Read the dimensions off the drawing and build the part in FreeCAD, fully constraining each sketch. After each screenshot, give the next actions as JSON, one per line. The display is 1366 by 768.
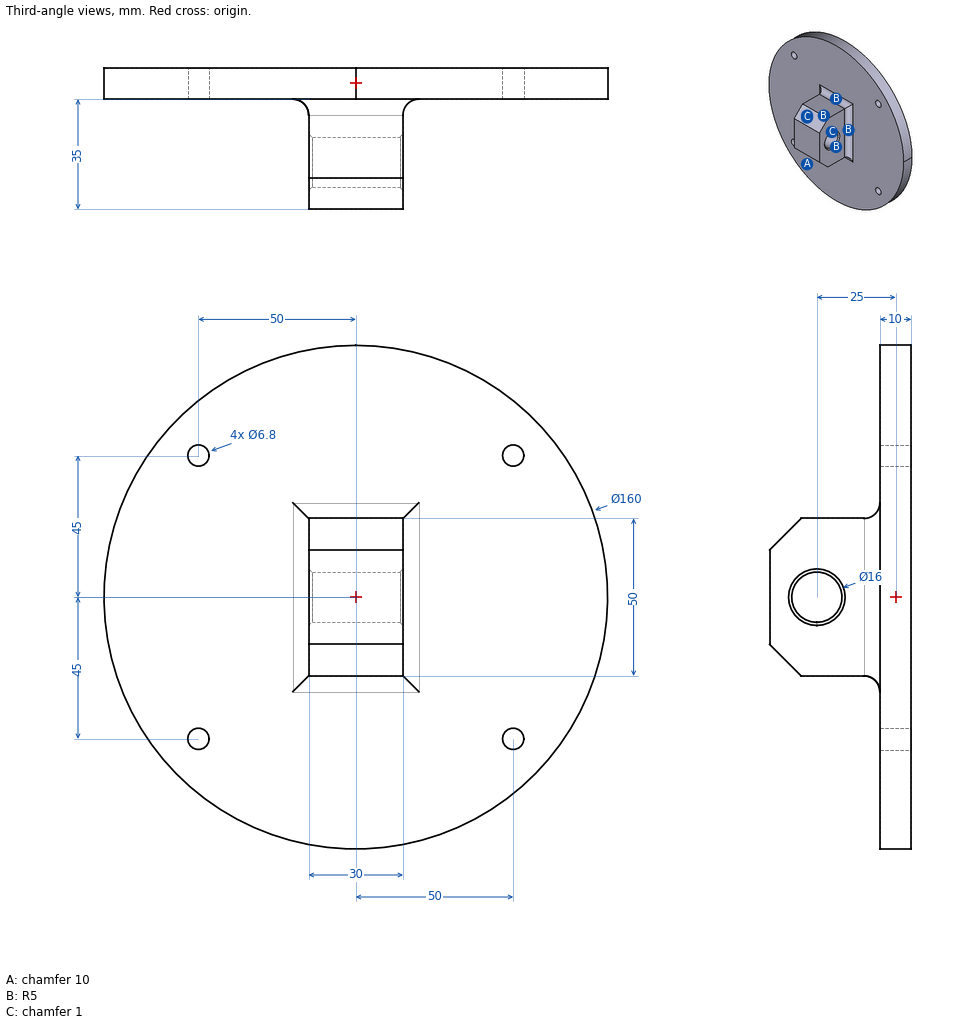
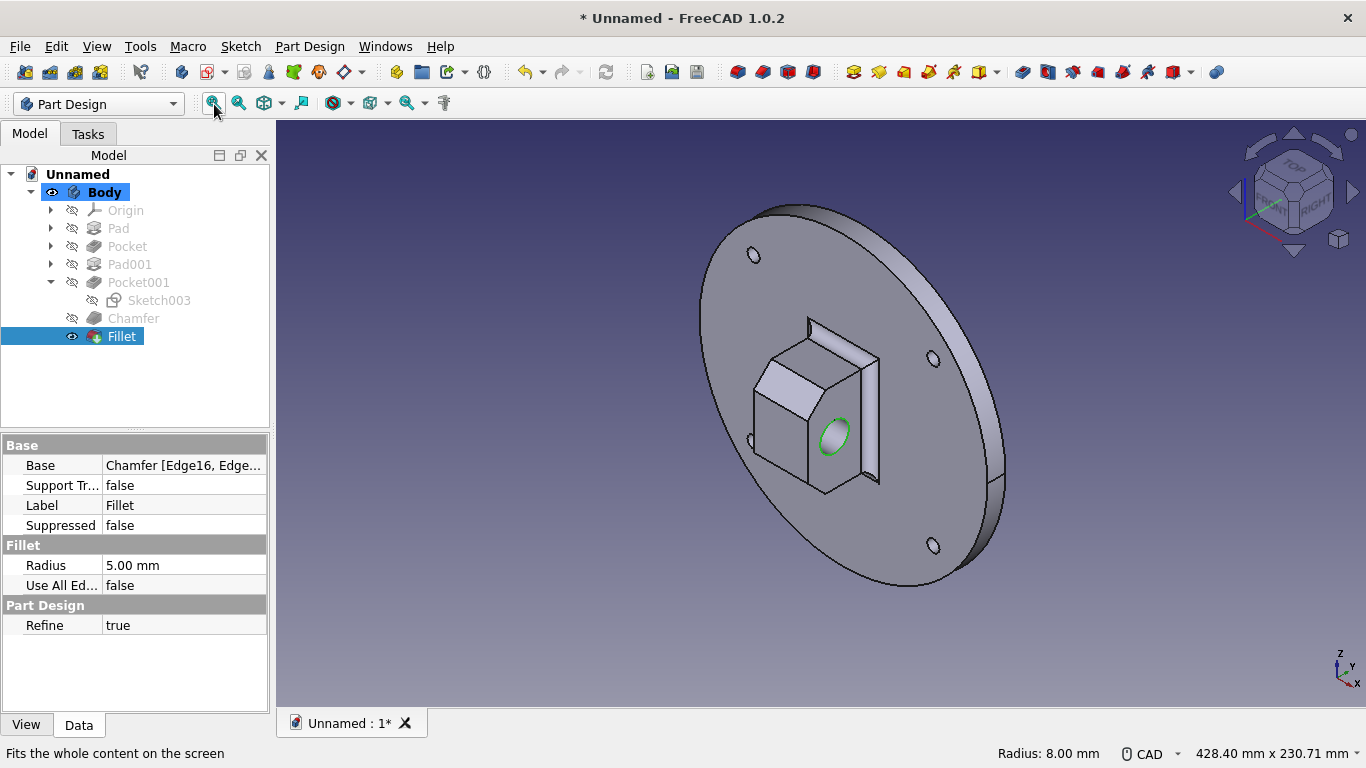
{"action": "key", "text": "1"}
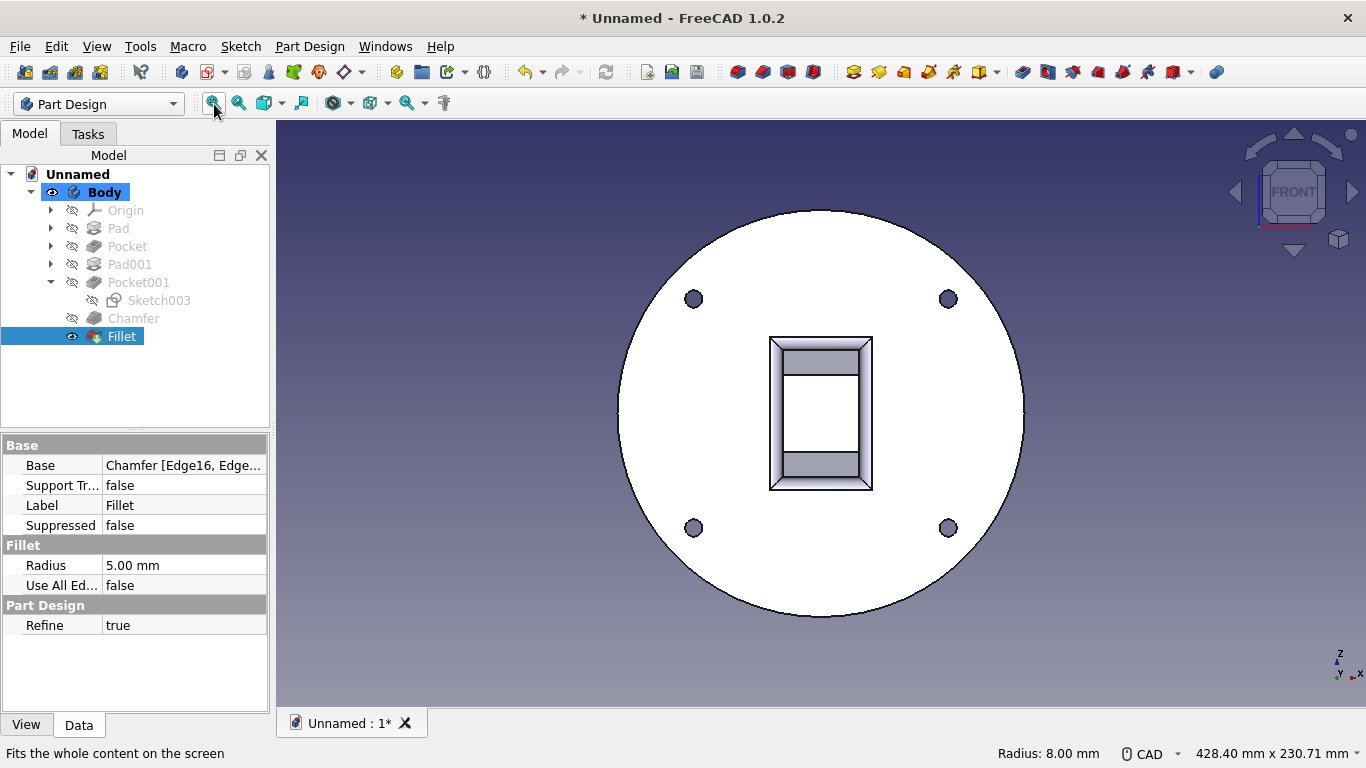
{"action": "key", "text": "3"}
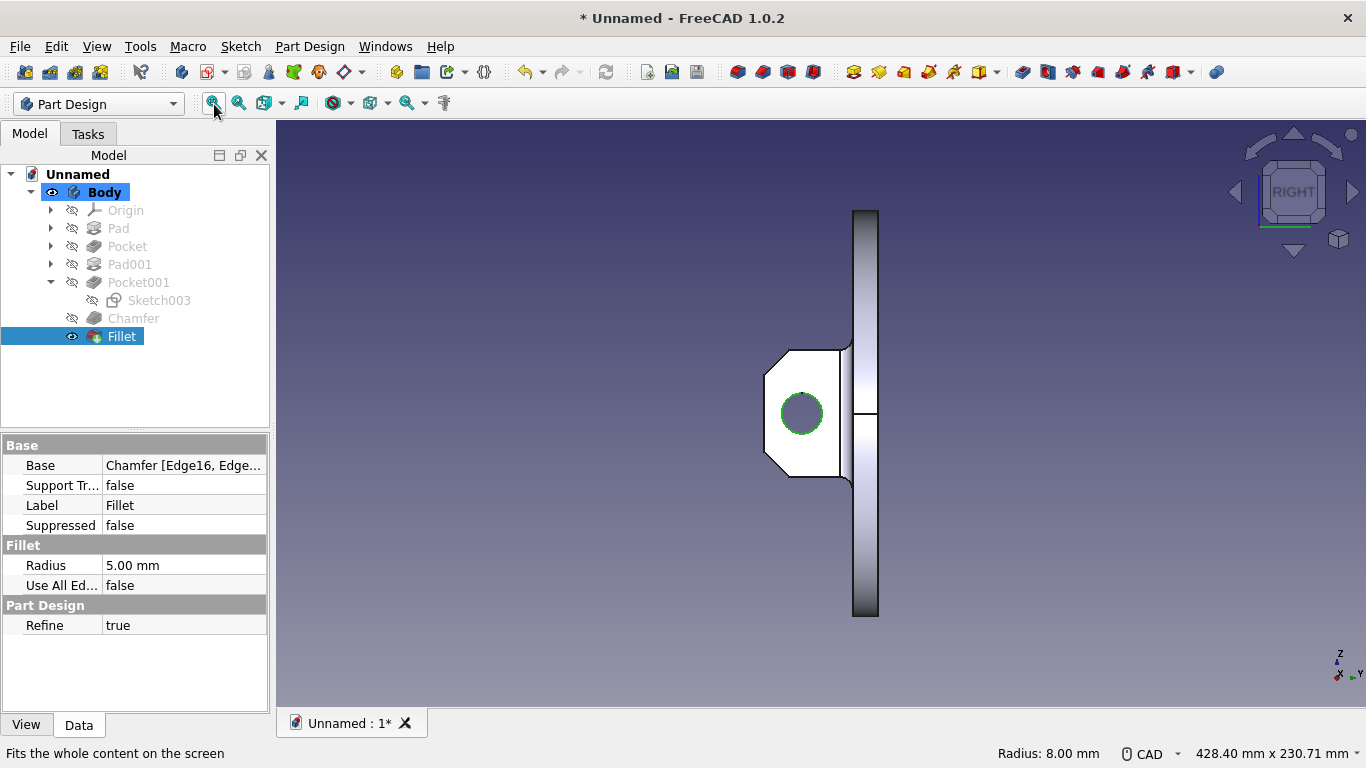
{"action": "key", "text": "5"}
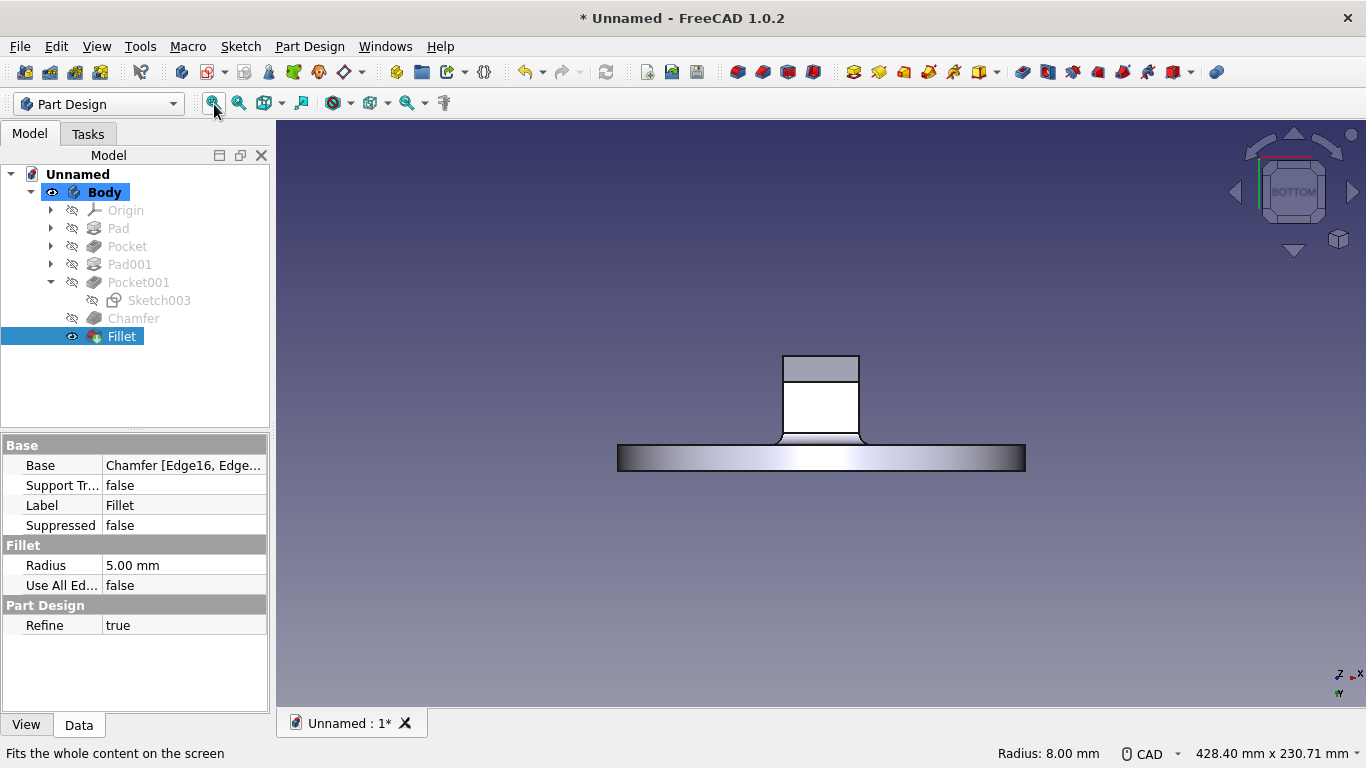
{"action": "left_click", "coordinate": [214, 104]}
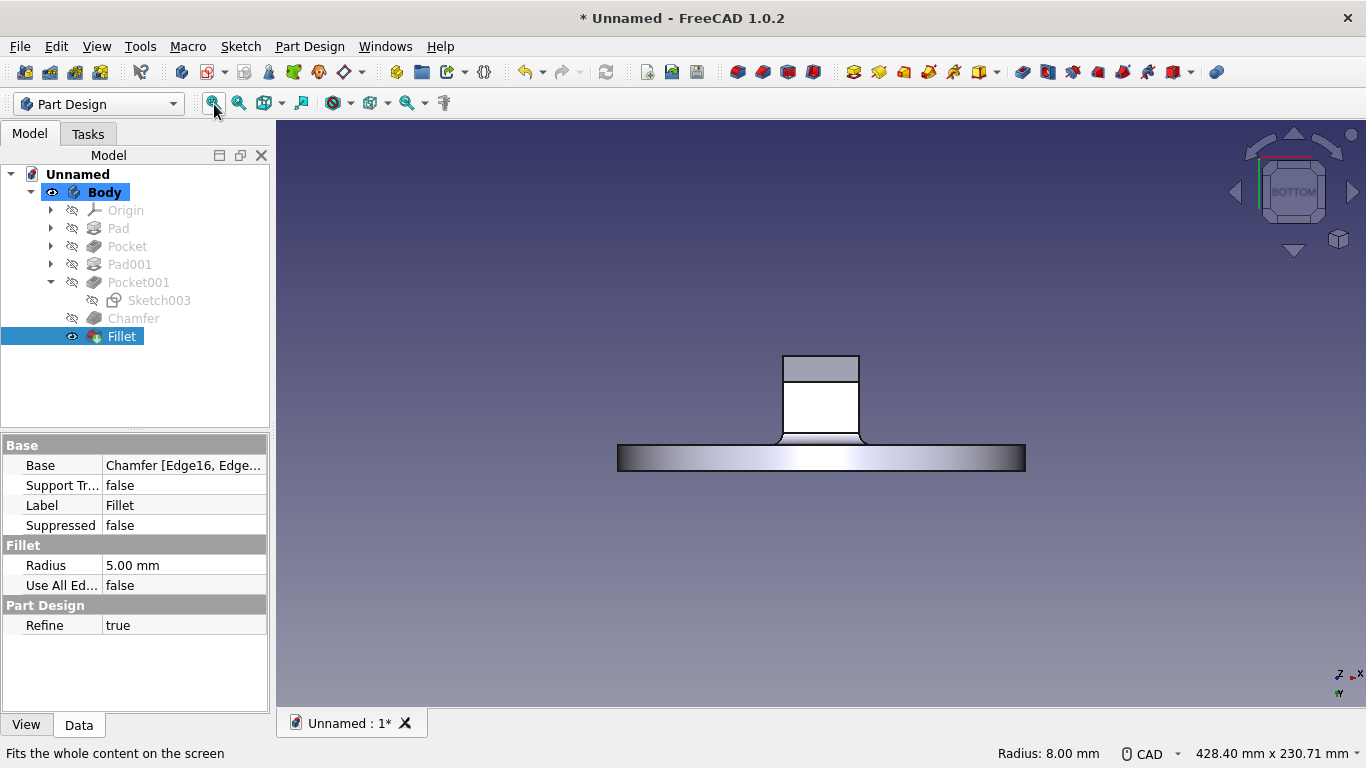
{"action": "key", "text": "4"}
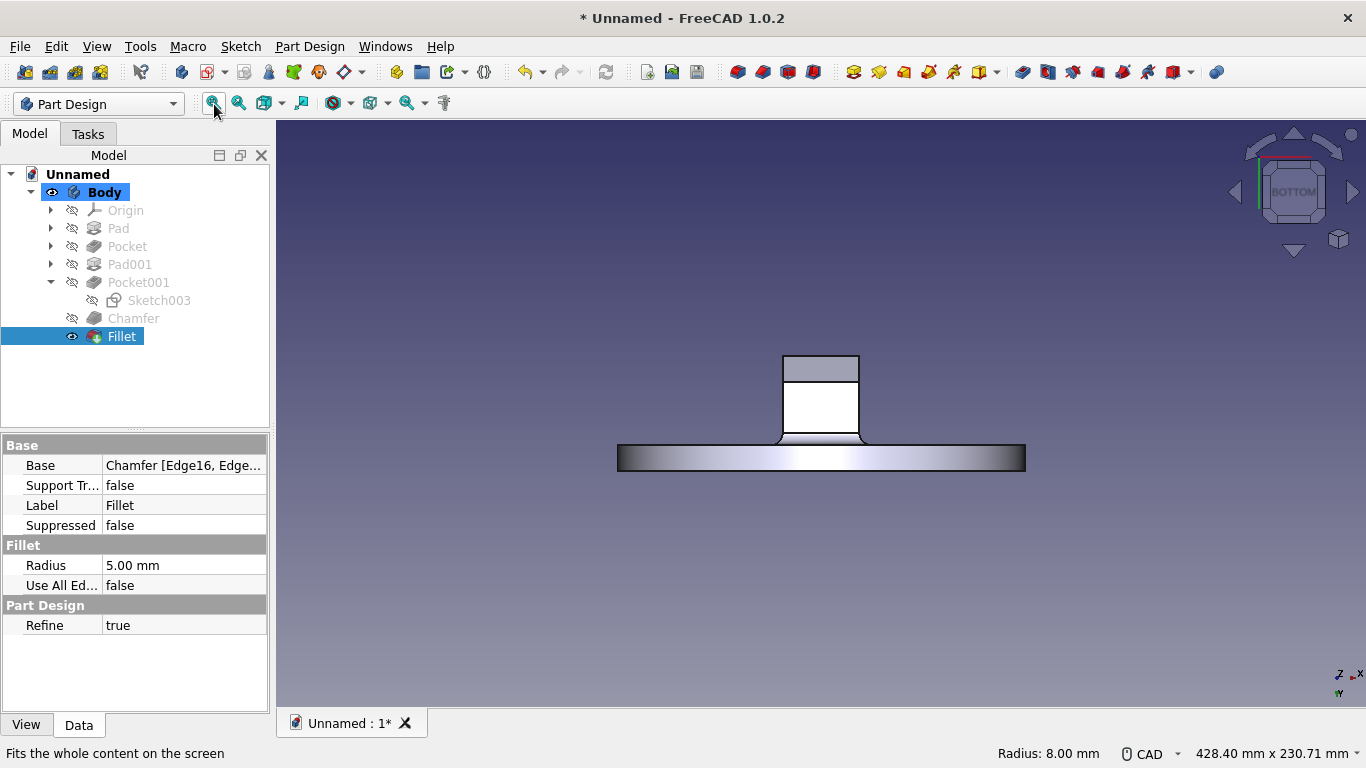
{"action": "key", "text": "6"}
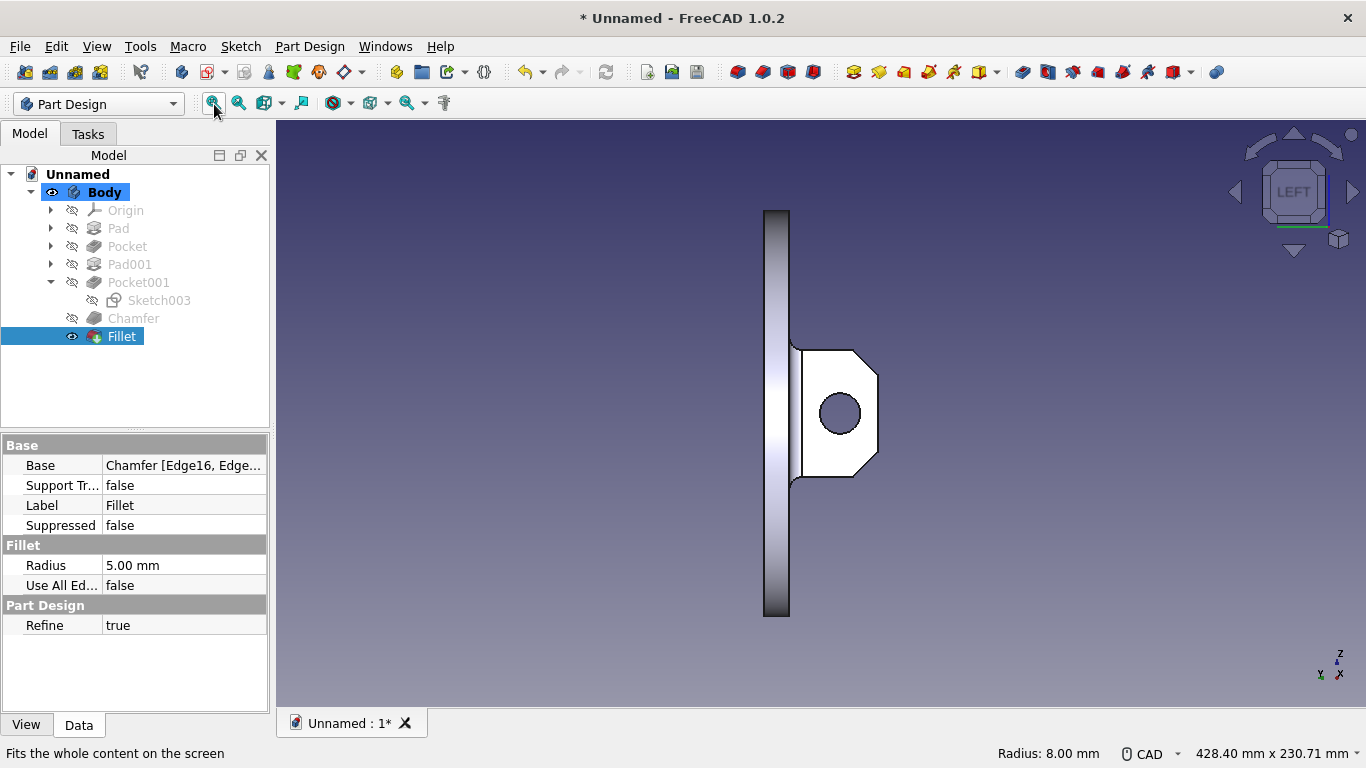
{"action": "left_click", "coordinate": [840, 433], "text": "ctrl"}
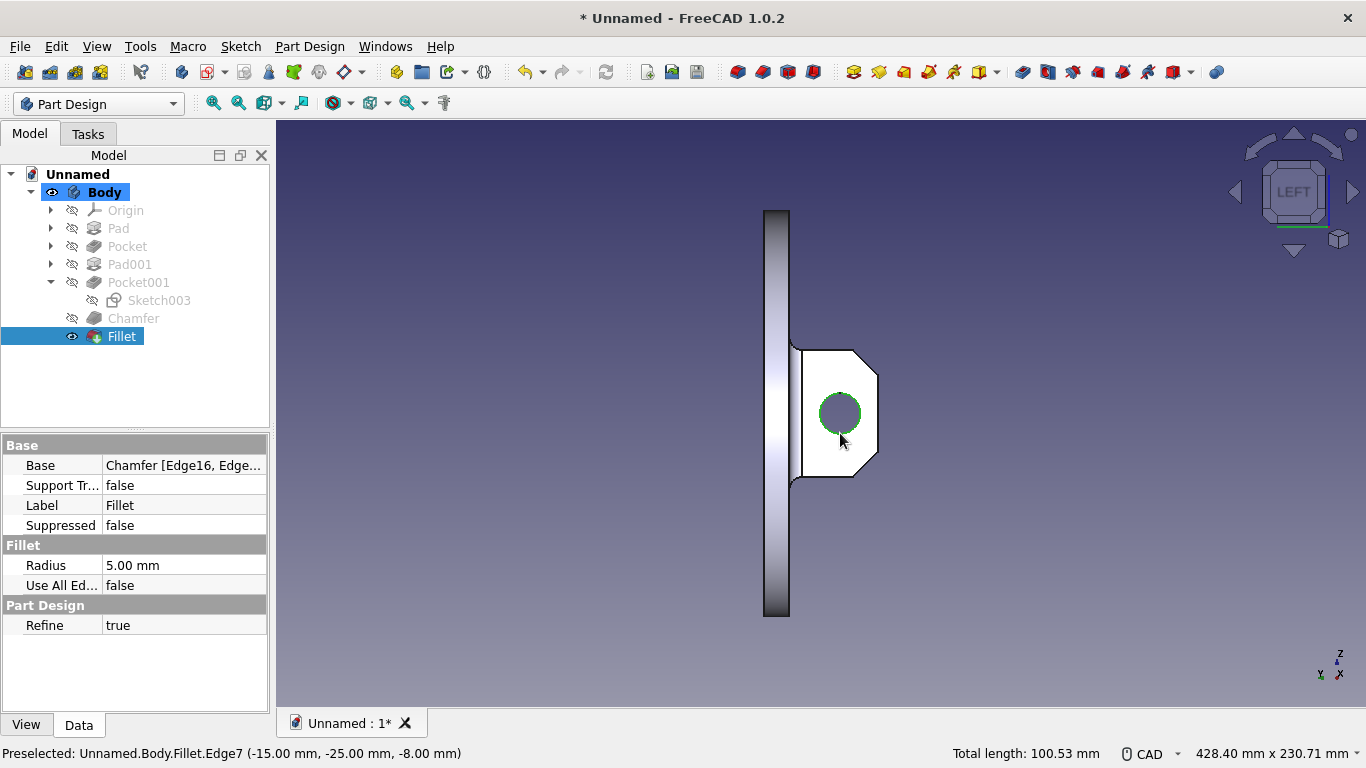
{"action": "left_click", "coordinate": [763, 72]}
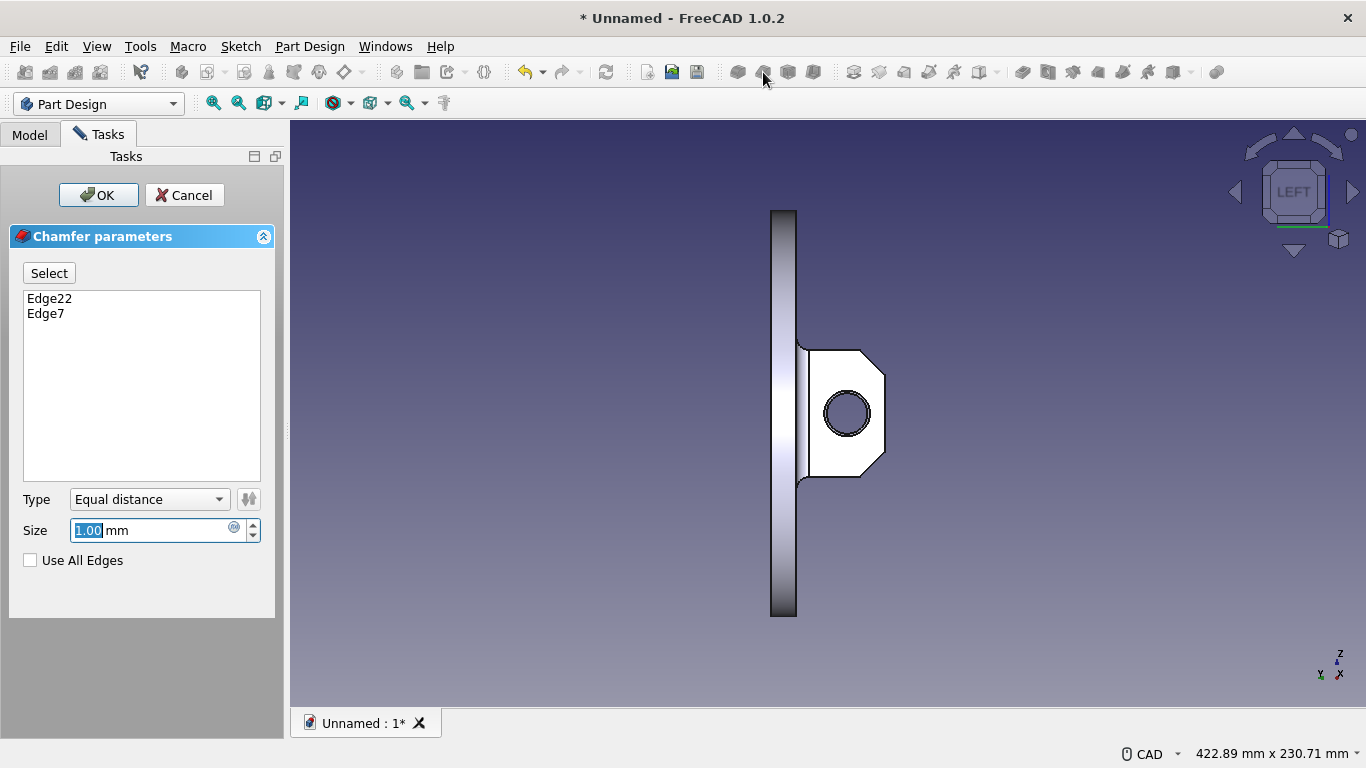
{"action": "type", "text": "1"}
{"action": "key", "text": "Tab"}